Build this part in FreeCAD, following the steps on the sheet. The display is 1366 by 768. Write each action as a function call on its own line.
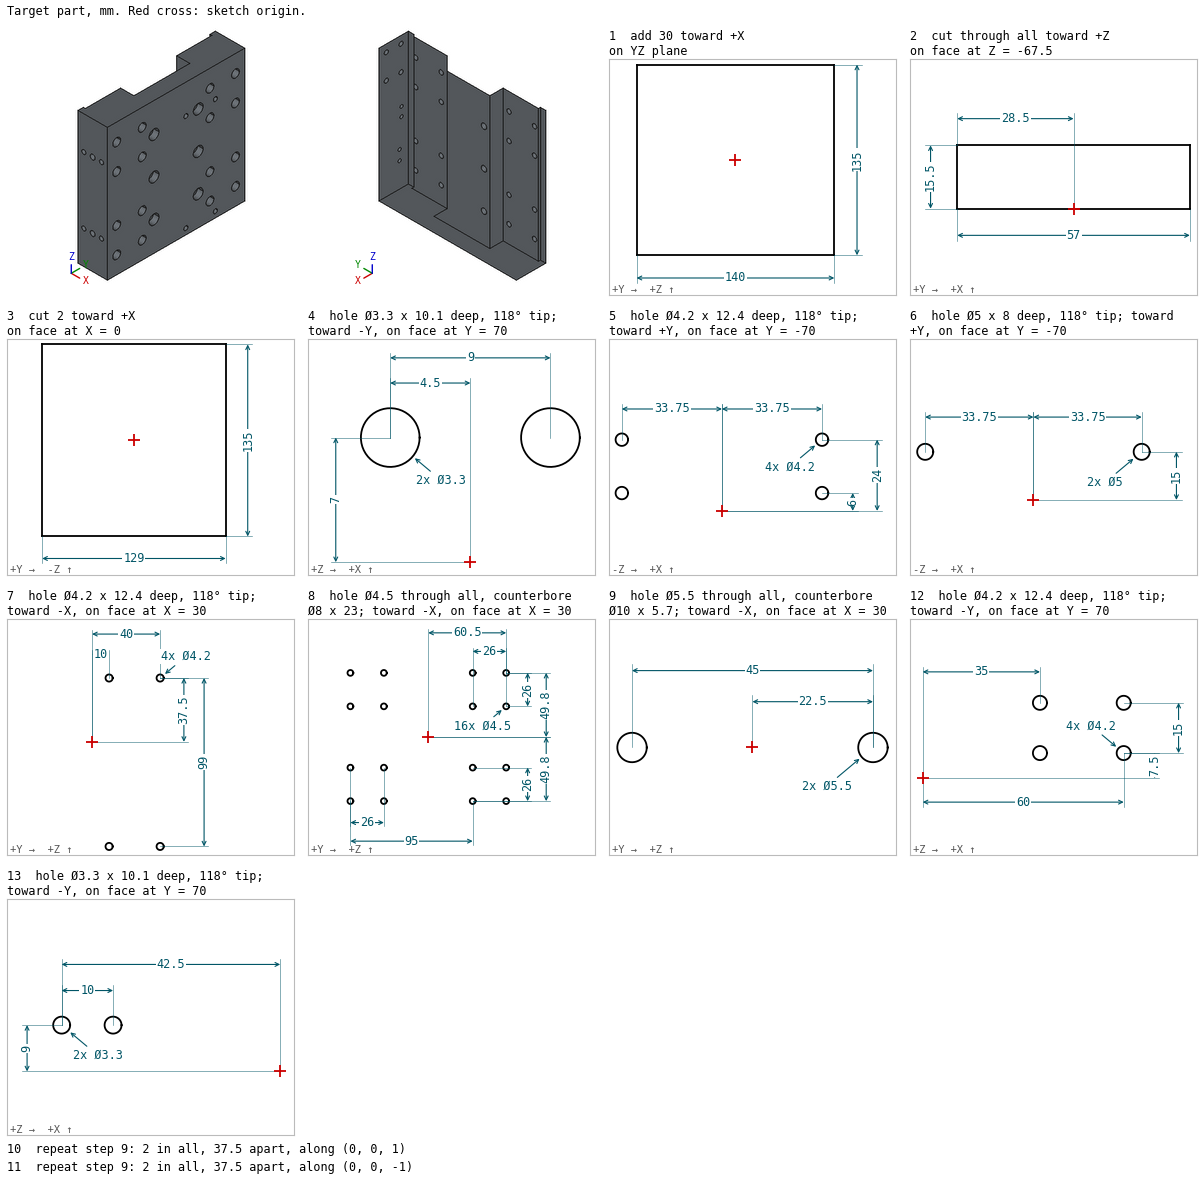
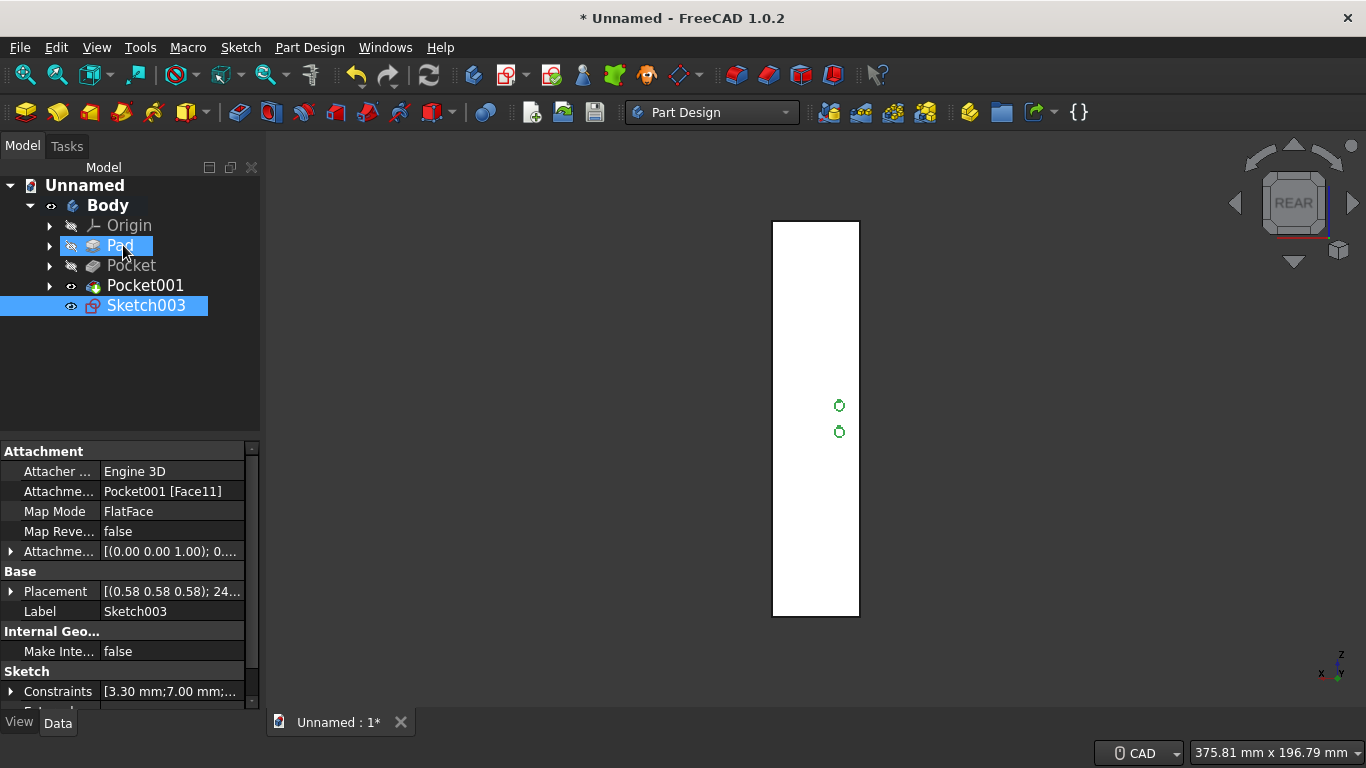
click(272, 112)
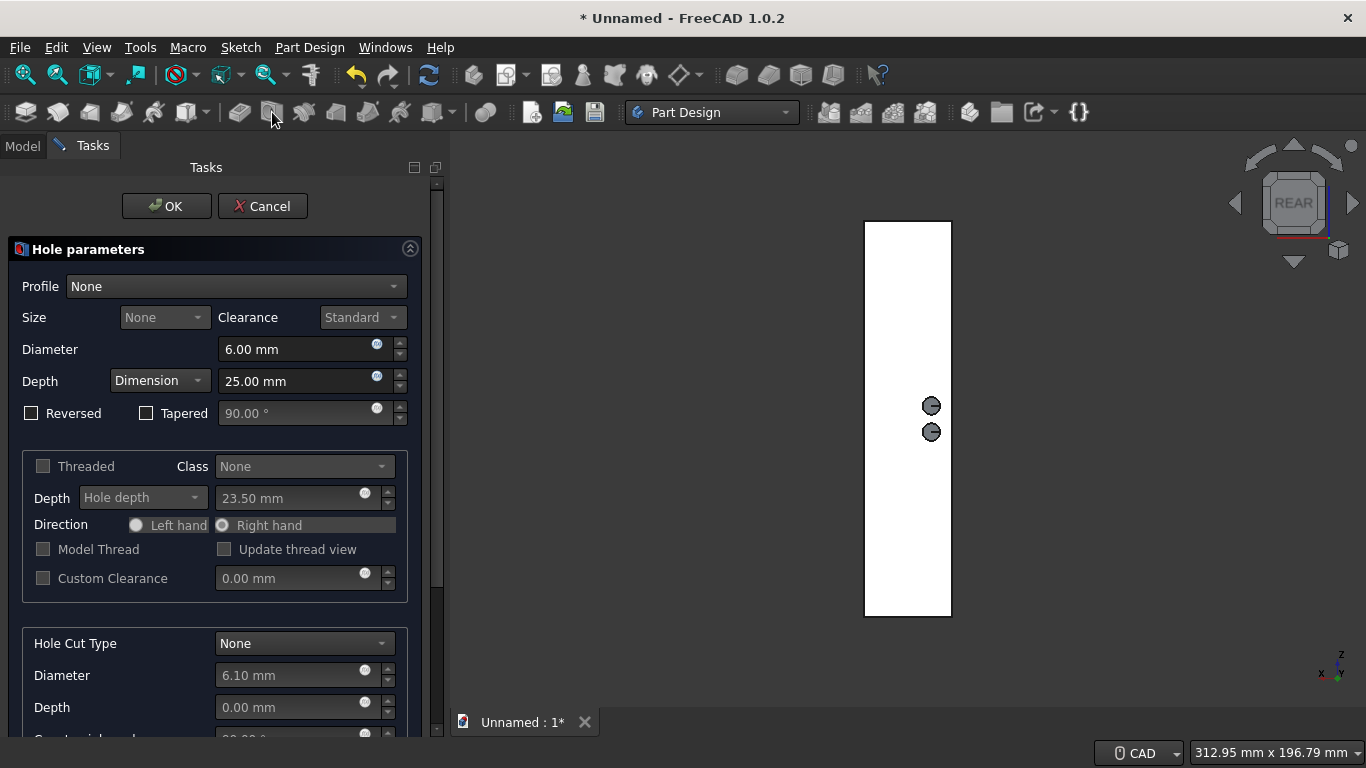
triple_click(305, 349)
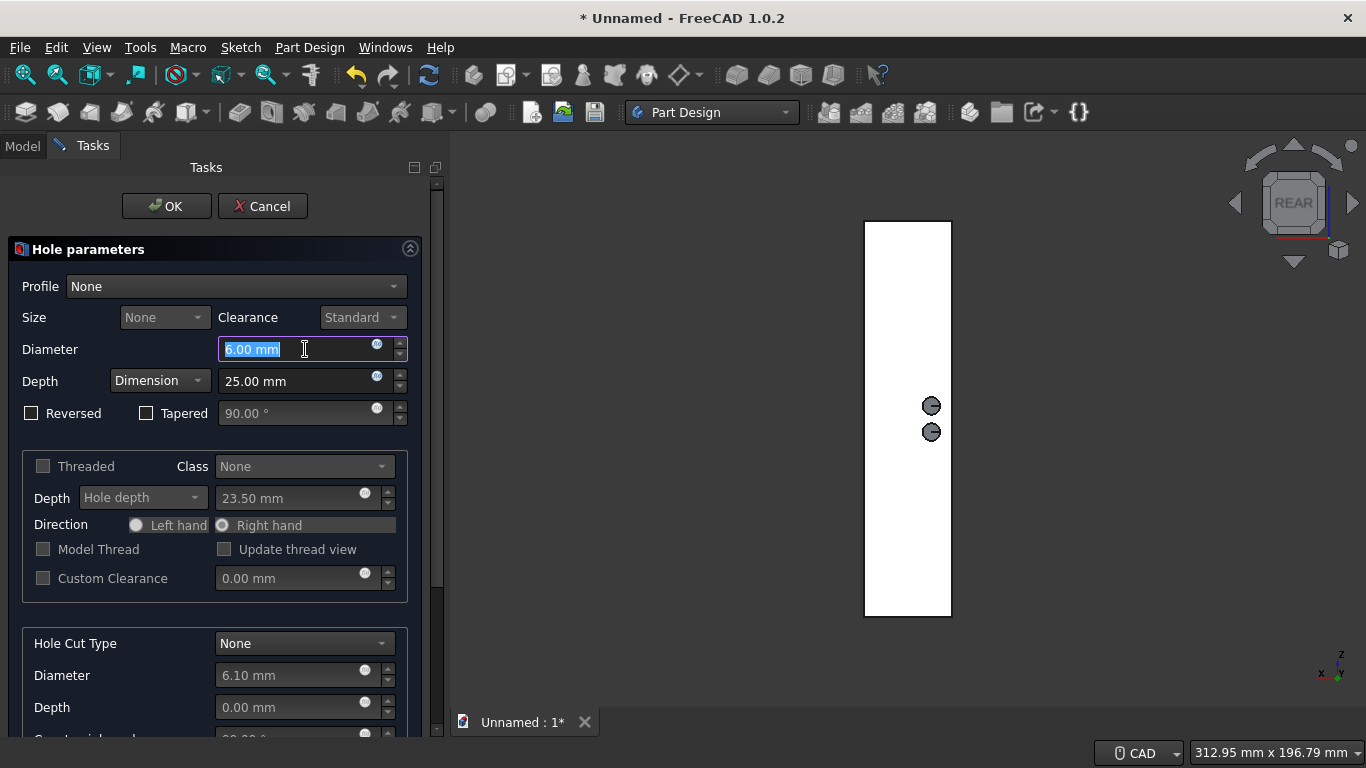
text(3.3)
key(Tab)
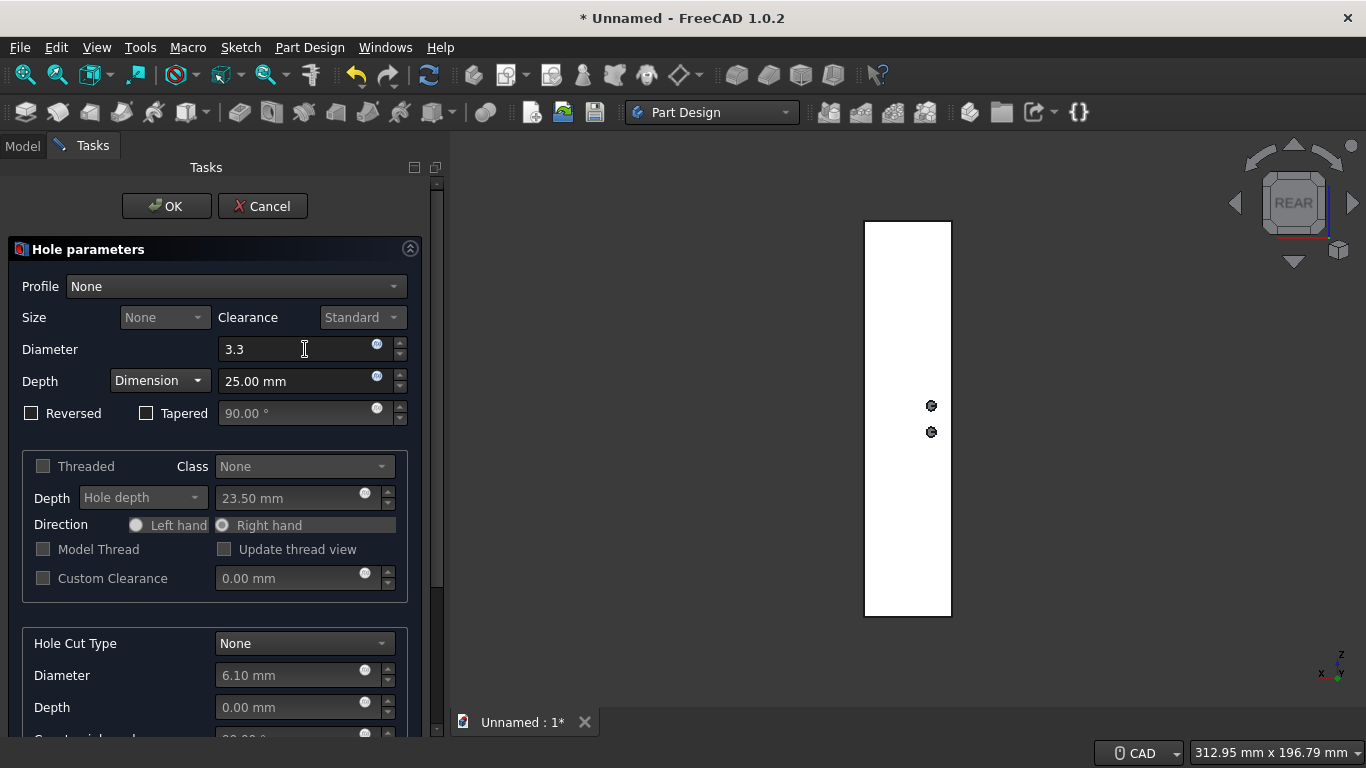
triple_click(305, 381)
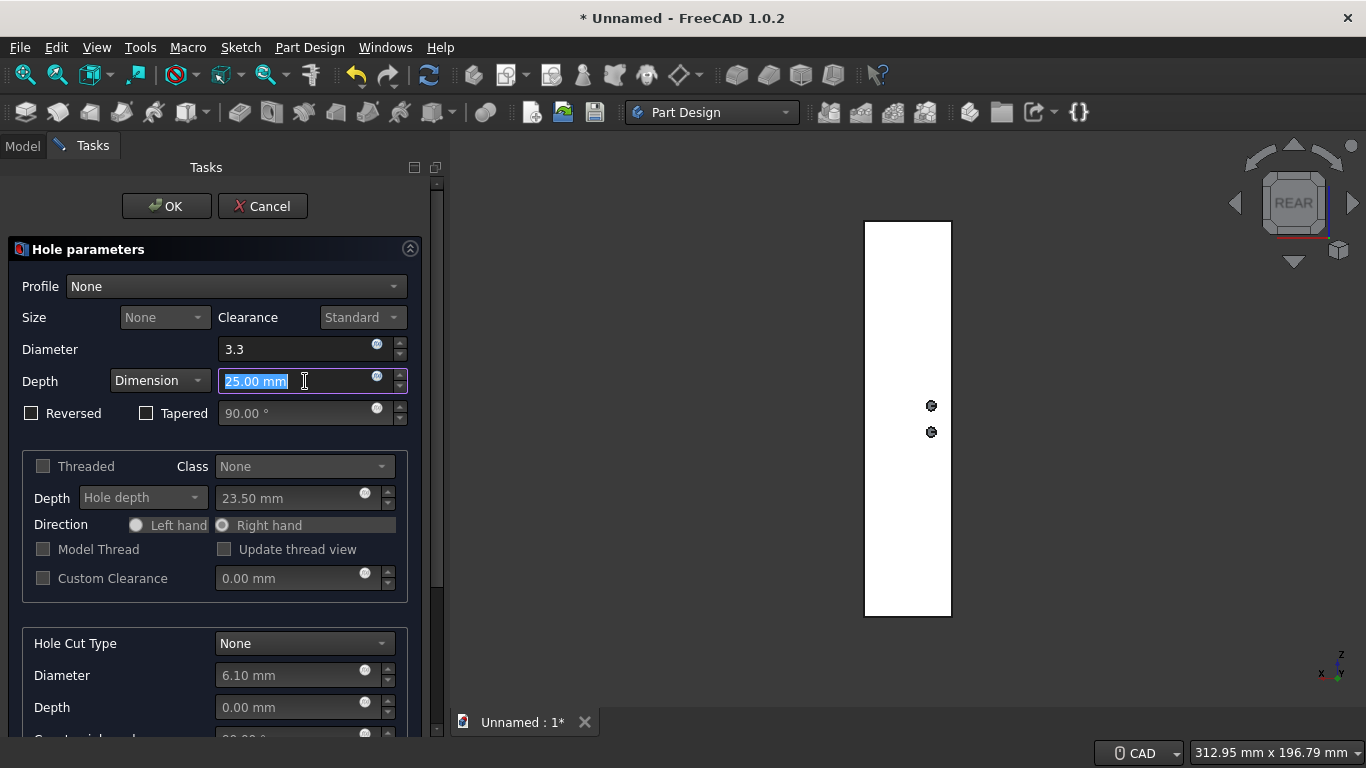
text(10.1)
key(Tab)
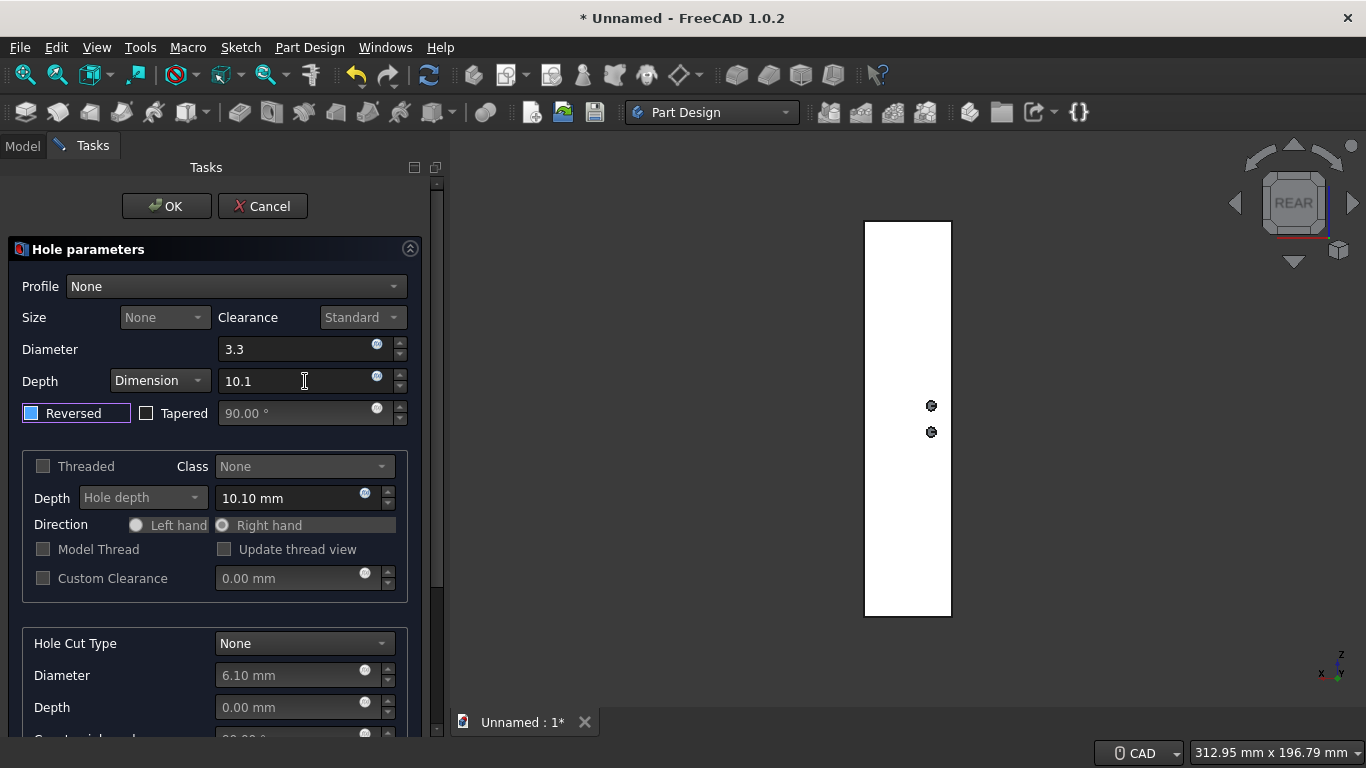
click(167, 206)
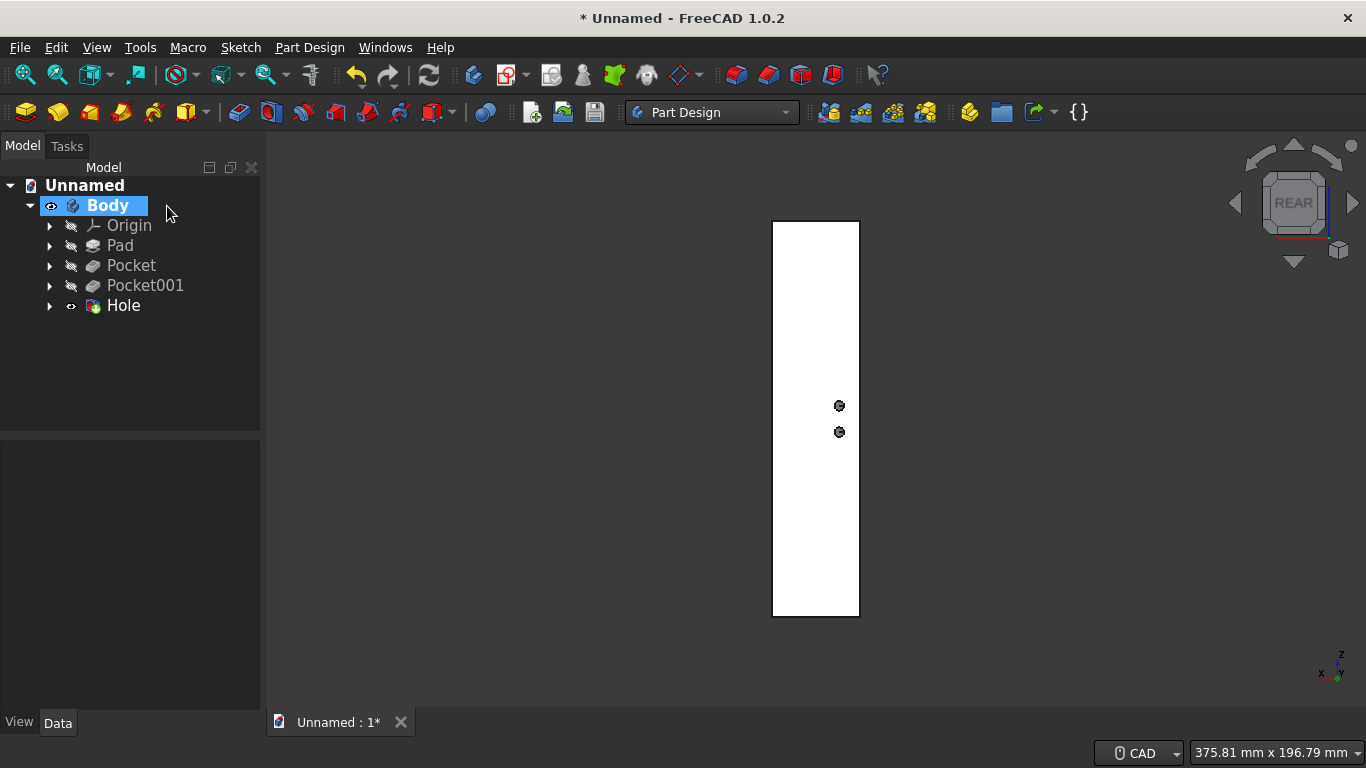
key(0)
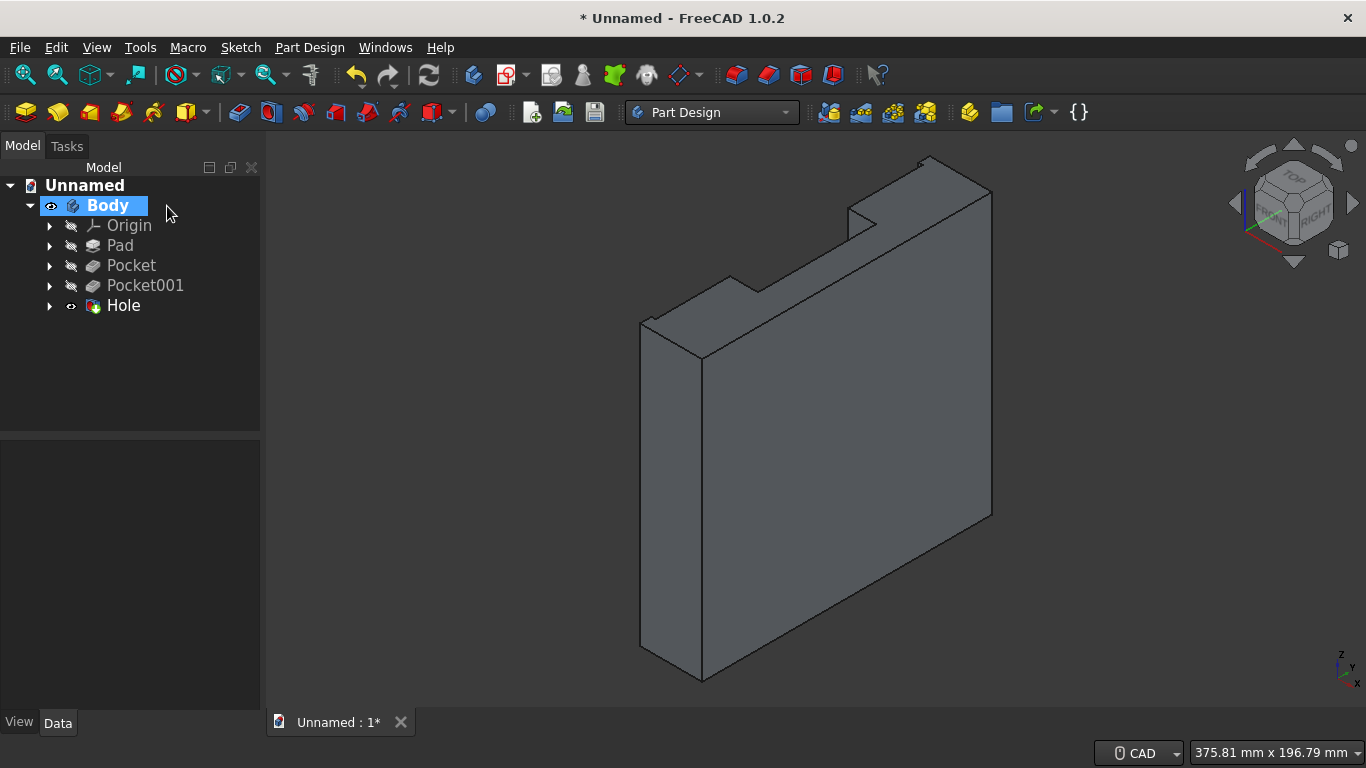
click(671, 548)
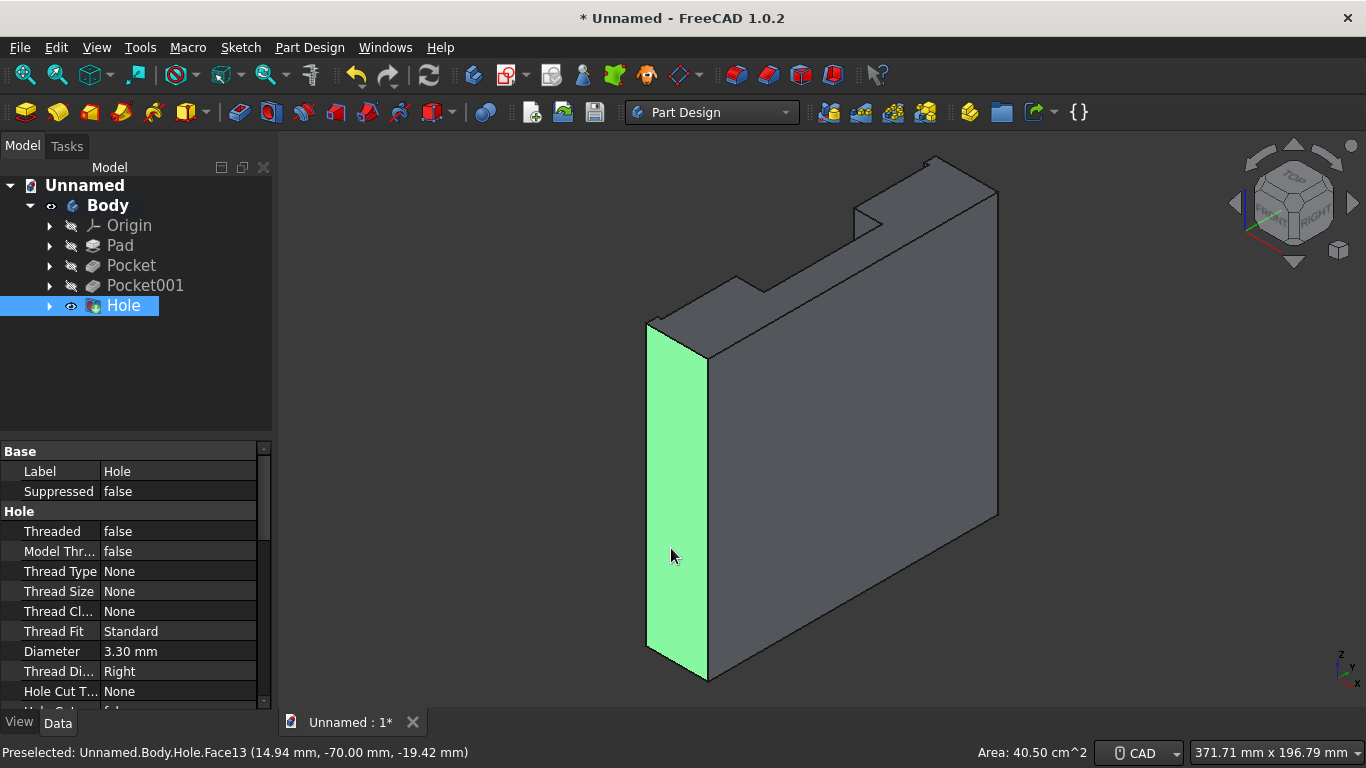
click(506, 76)